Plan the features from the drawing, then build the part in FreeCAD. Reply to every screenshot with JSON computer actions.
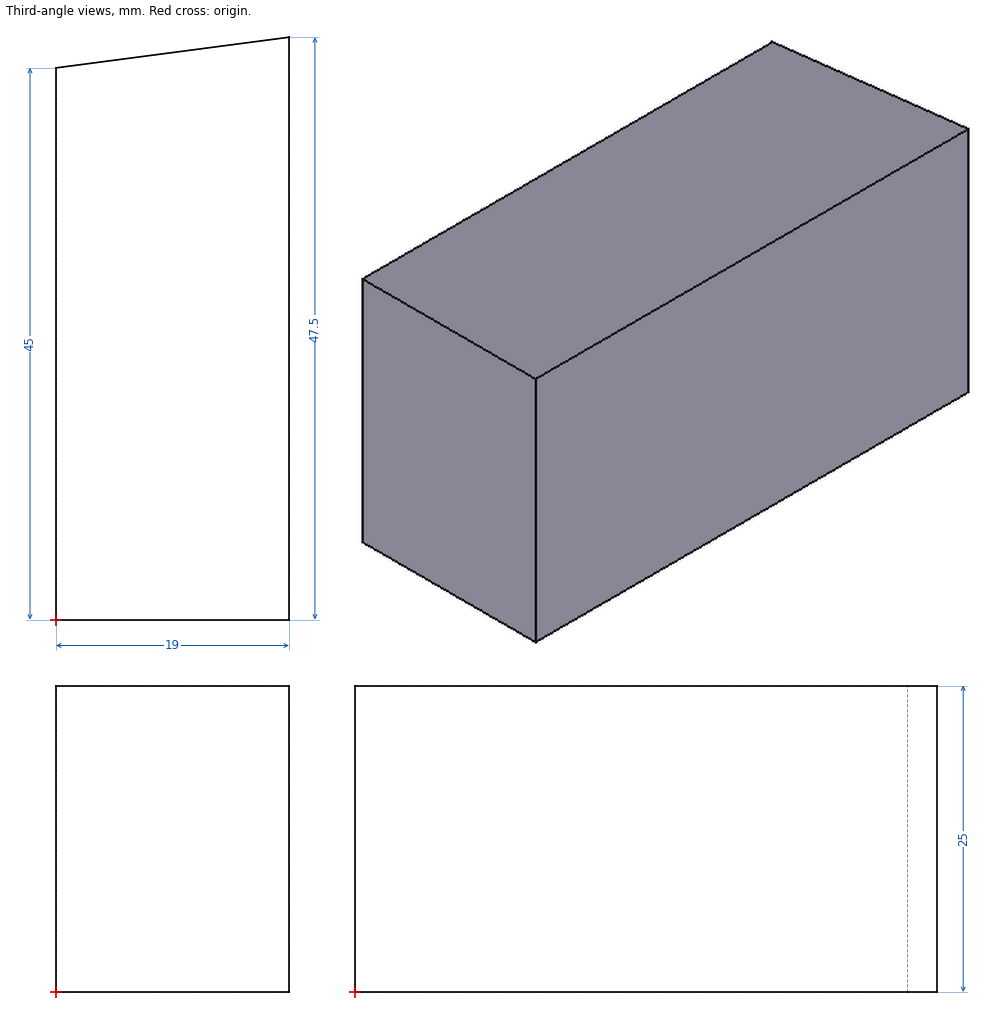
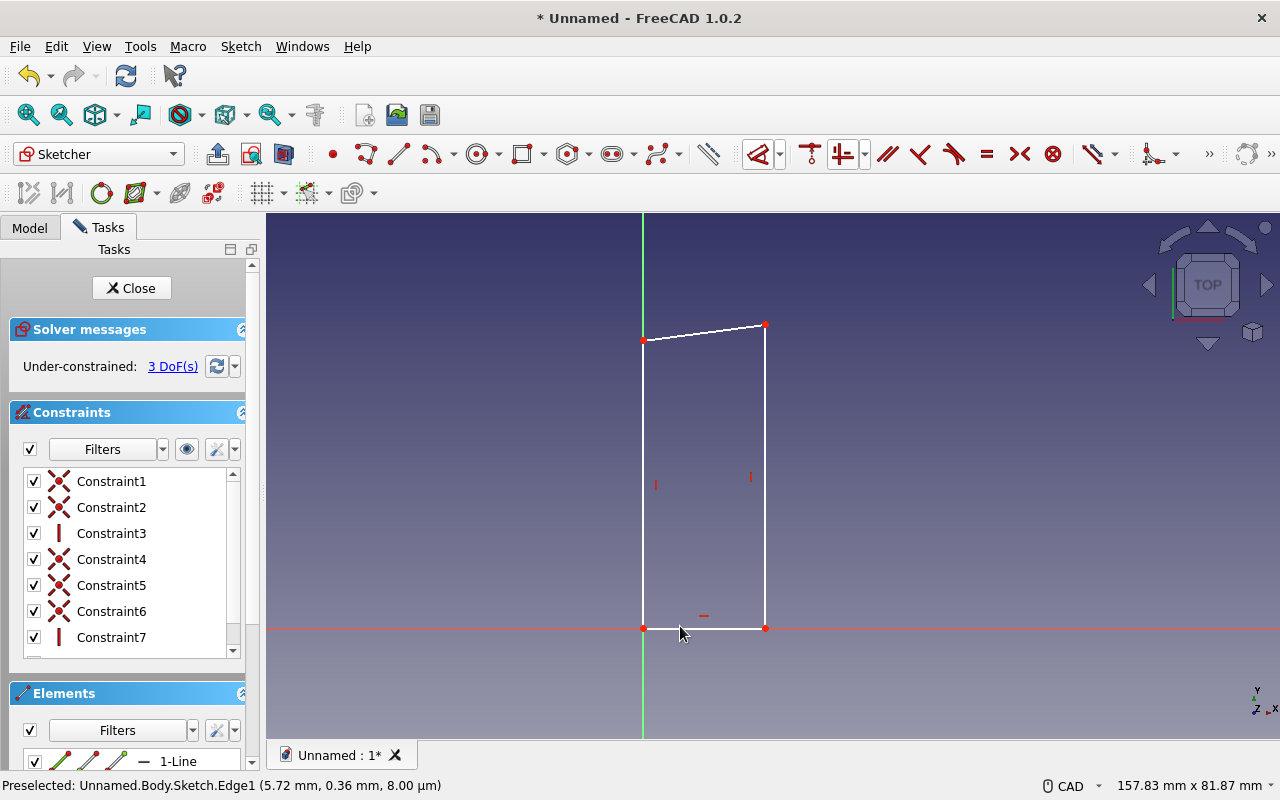
{"action": "left_click", "coordinate": [680, 629]}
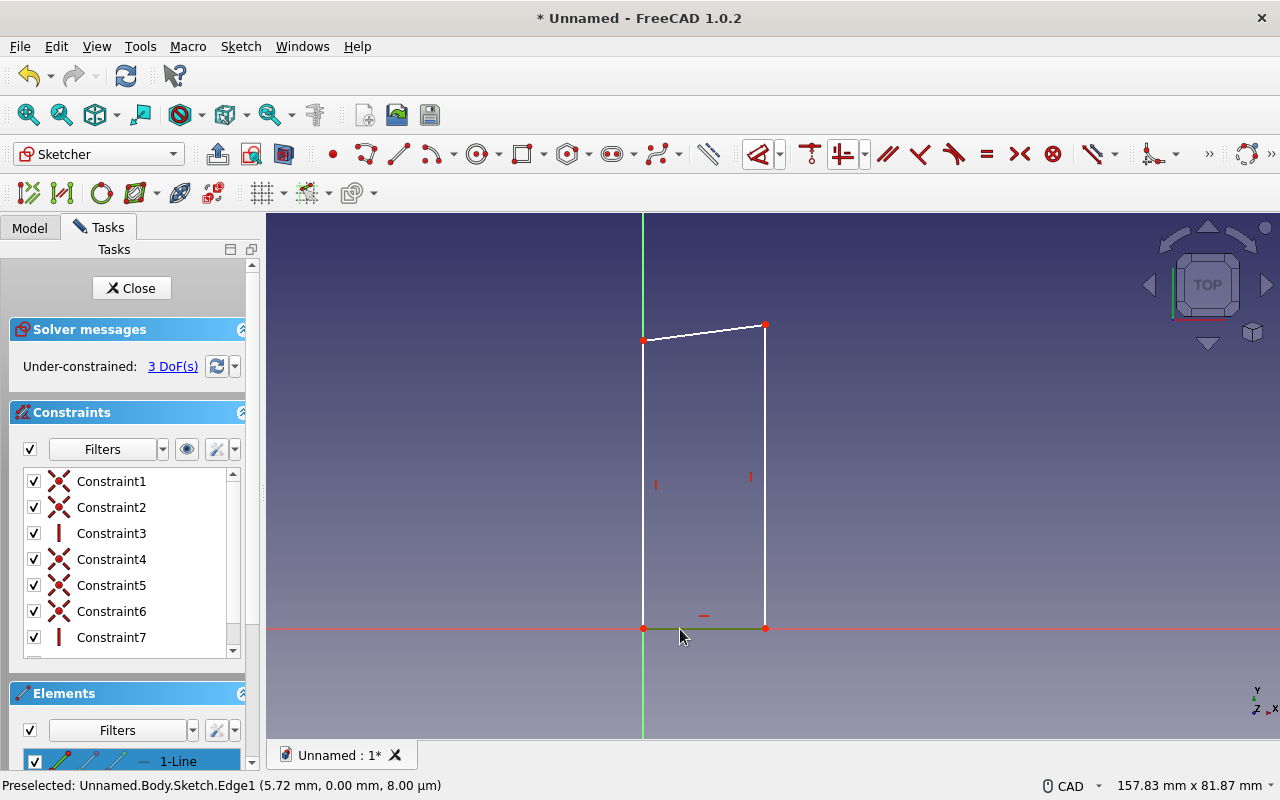
{"action": "key", "text": "l"}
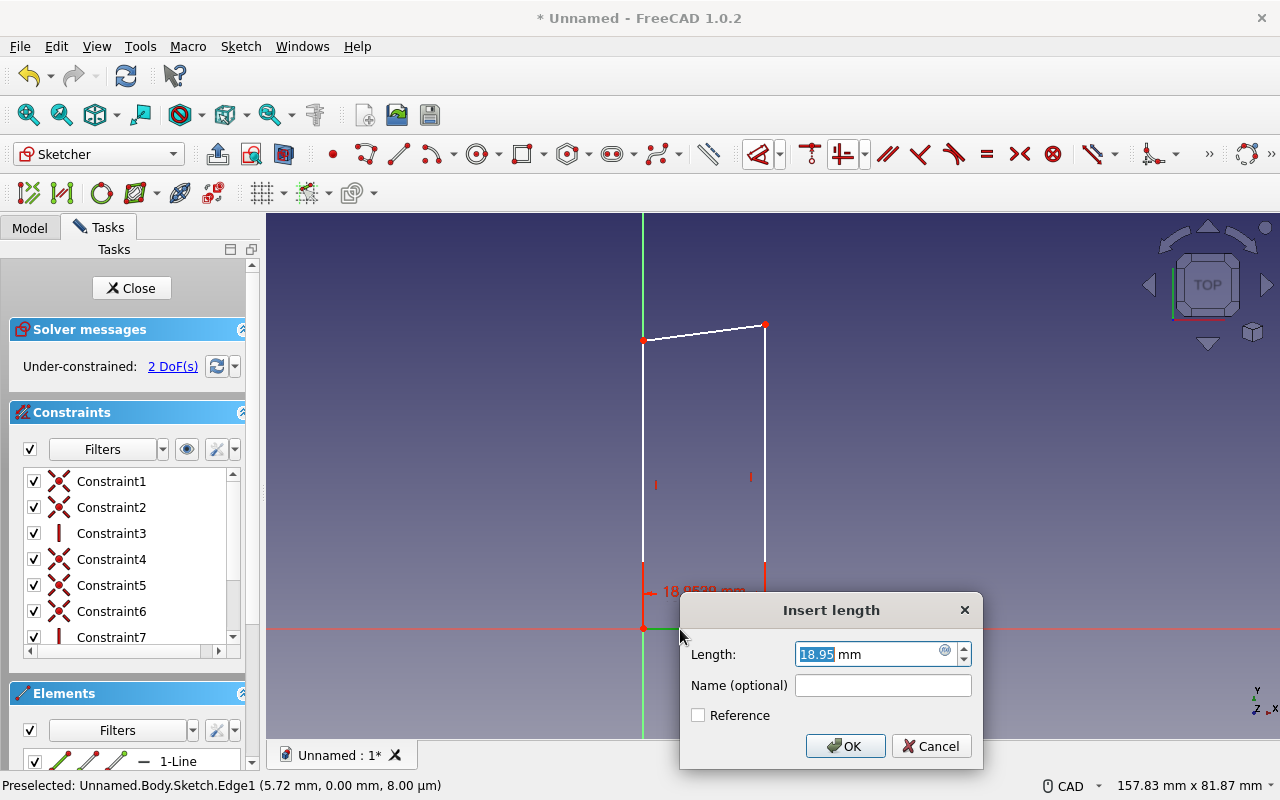
{"action": "type", "text": "19"}
{"action": "key", "text": "Return"}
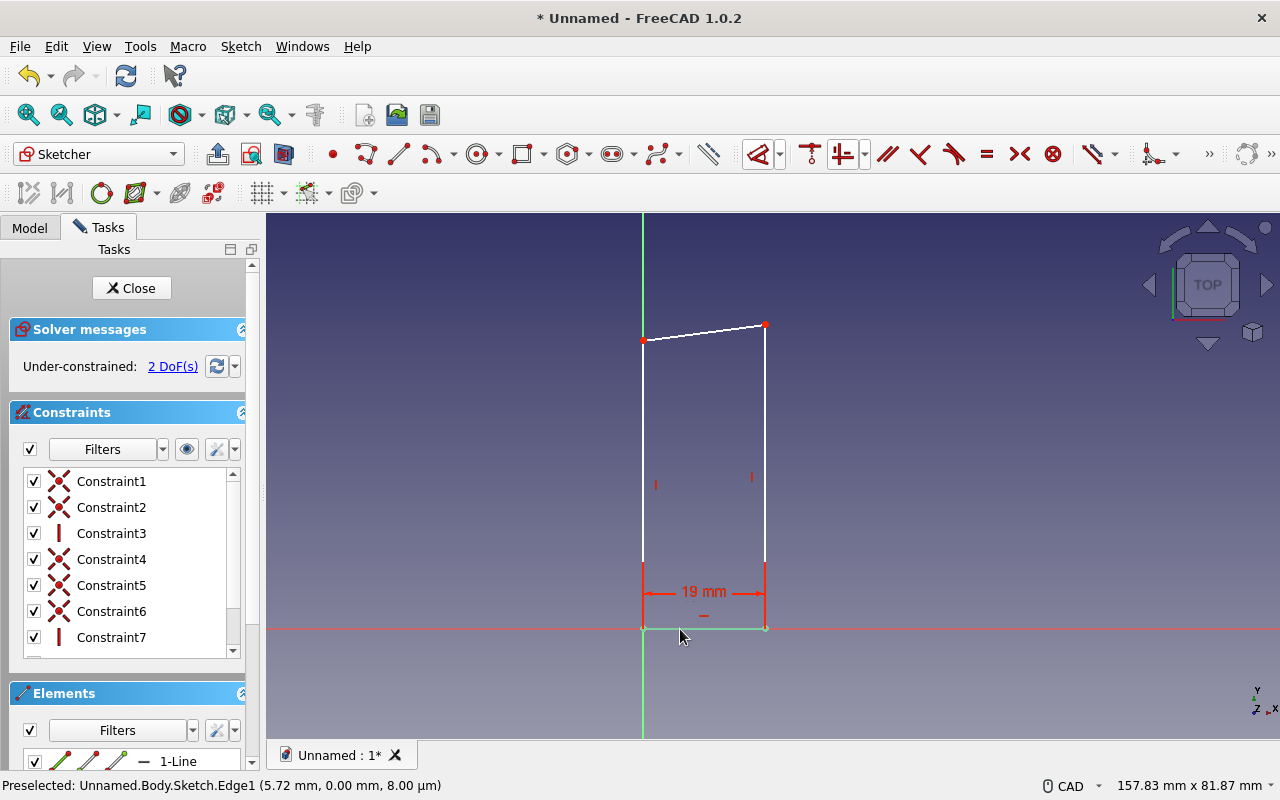
{"action": "left_click", "coordinate": [643, 427]}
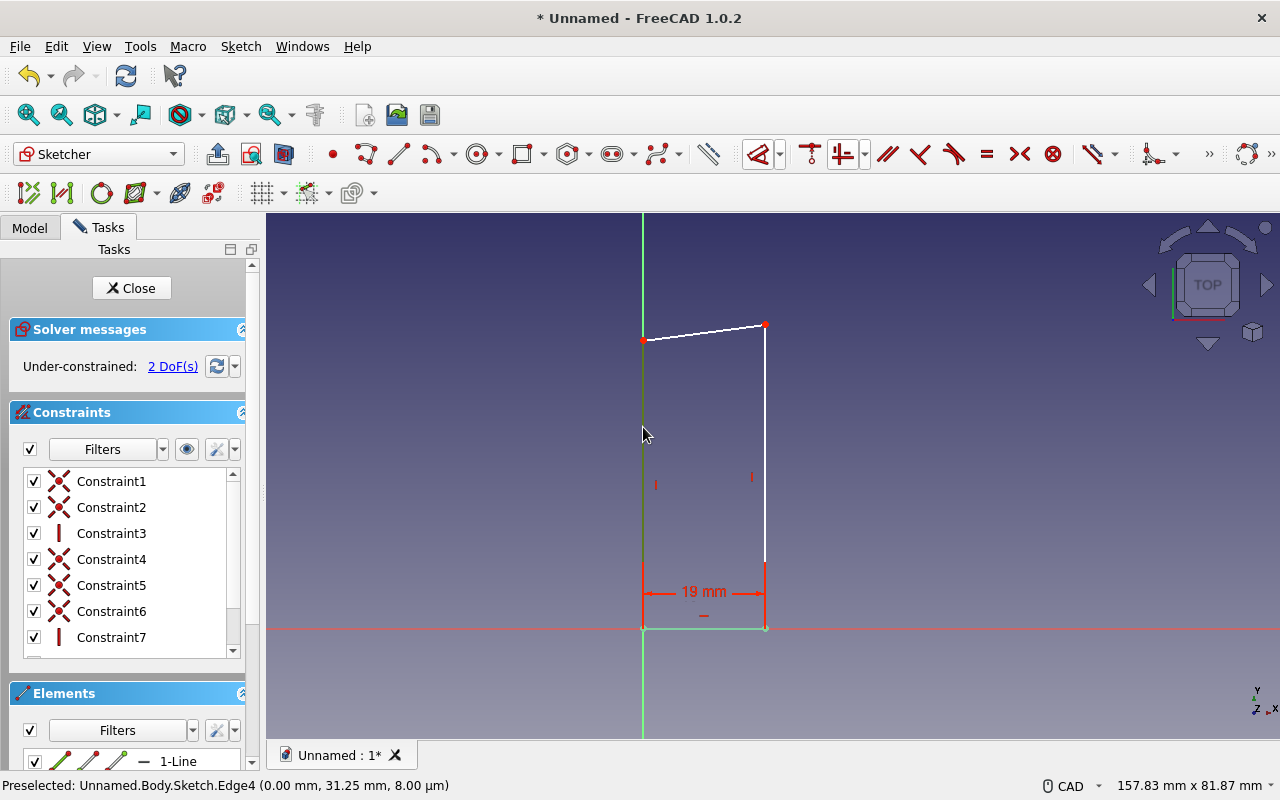
{"action": "key", "text": "i"}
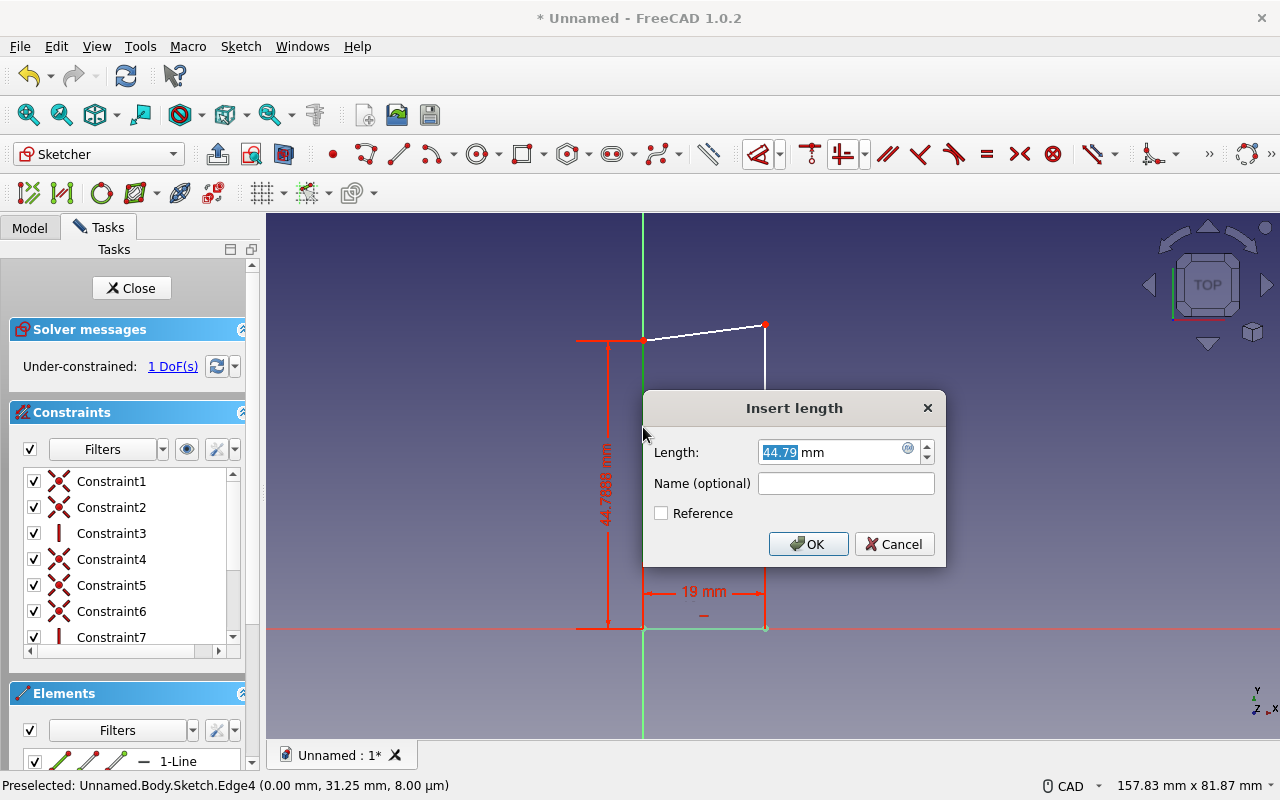
{"action": "type", "text": "45"}
{"action": "key", "text": "Return"}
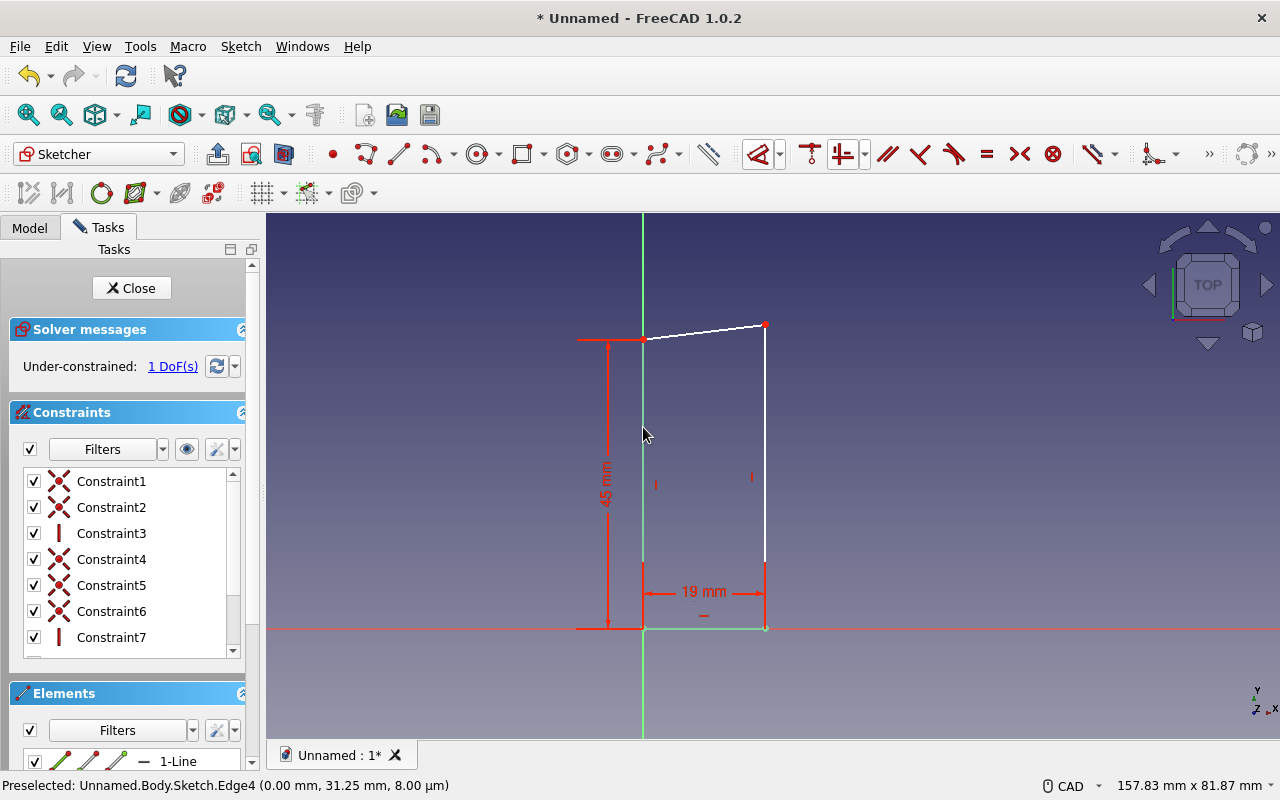
{"action": "left_click", "coordinate": [765, 538]}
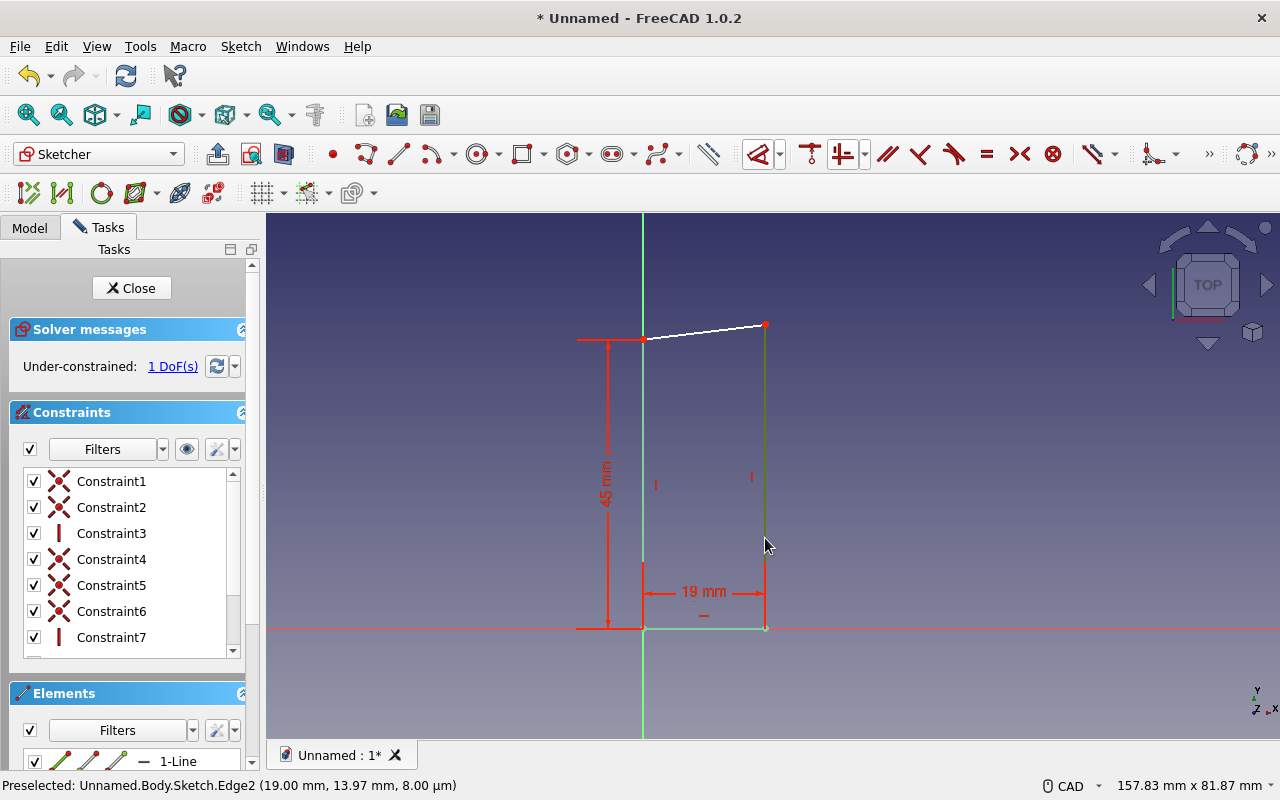
{"action": "key", "text": "i"}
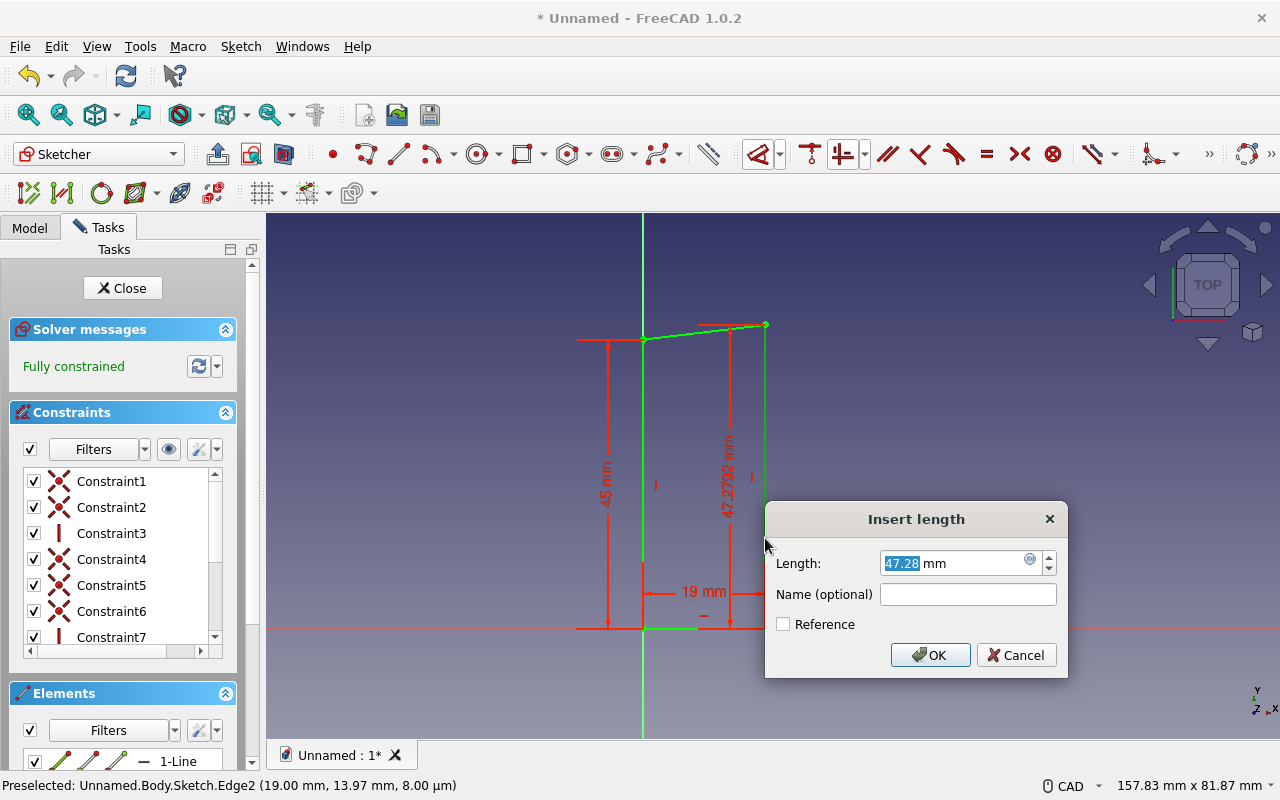
{"action": "type", "text": "47.5"}
{"action": "key", "text": "Return"}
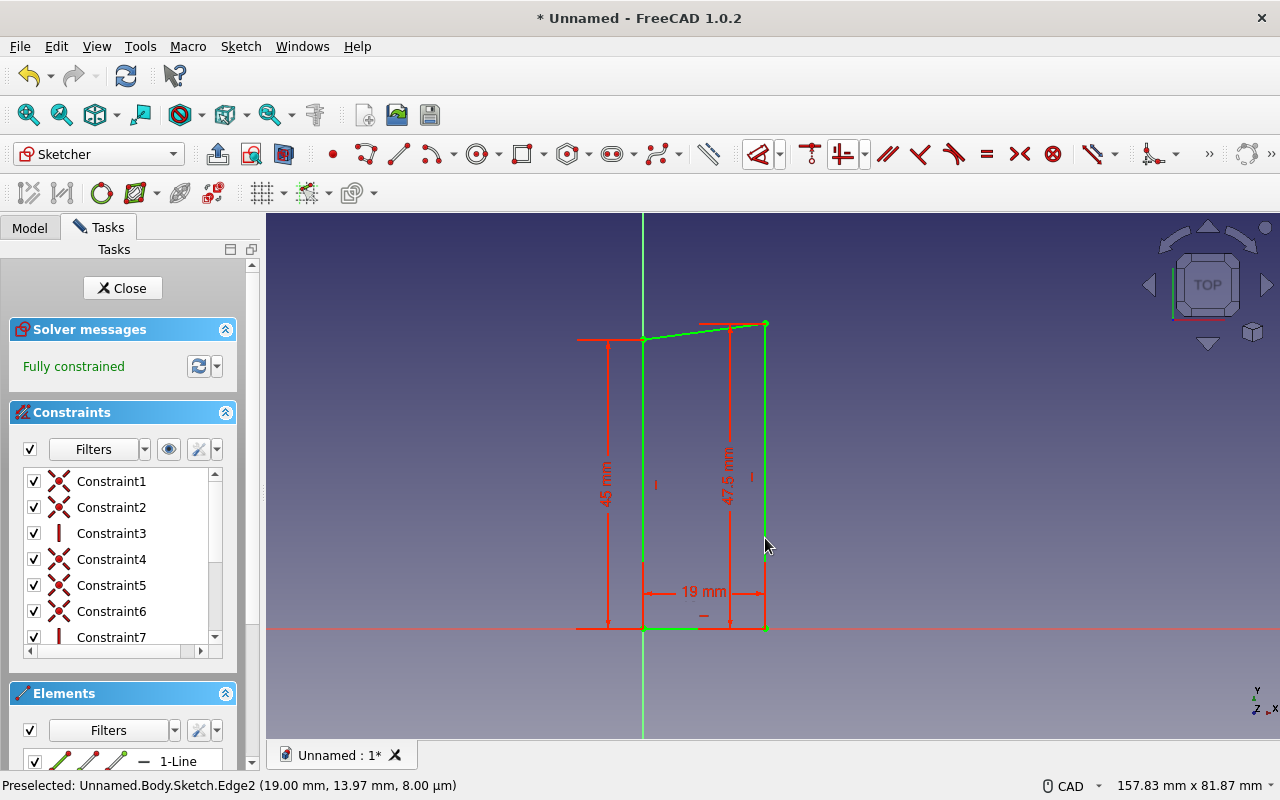
{"action": "left_click", "coordinate": [123, 288]}